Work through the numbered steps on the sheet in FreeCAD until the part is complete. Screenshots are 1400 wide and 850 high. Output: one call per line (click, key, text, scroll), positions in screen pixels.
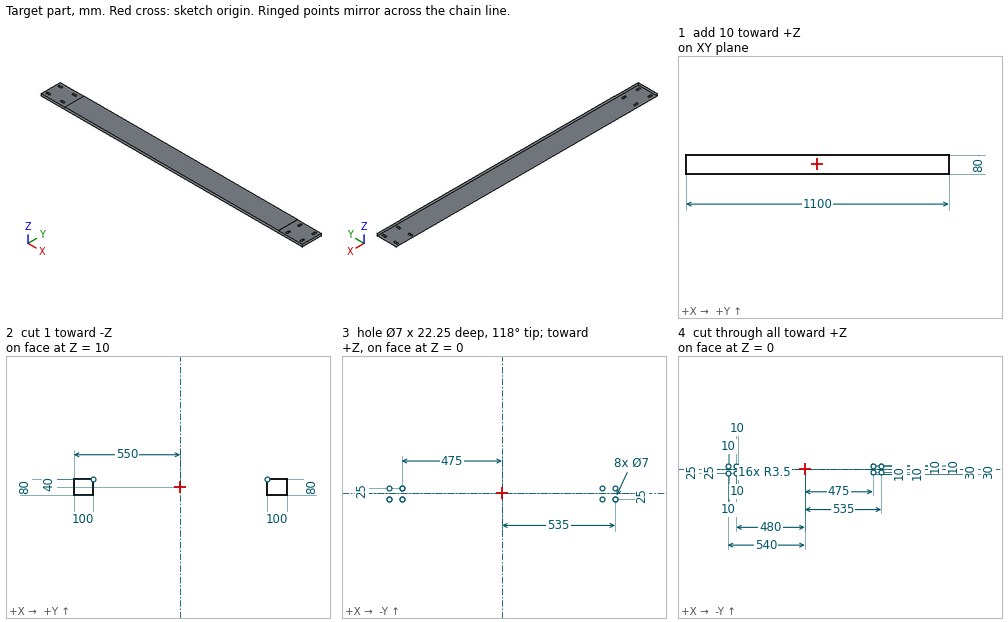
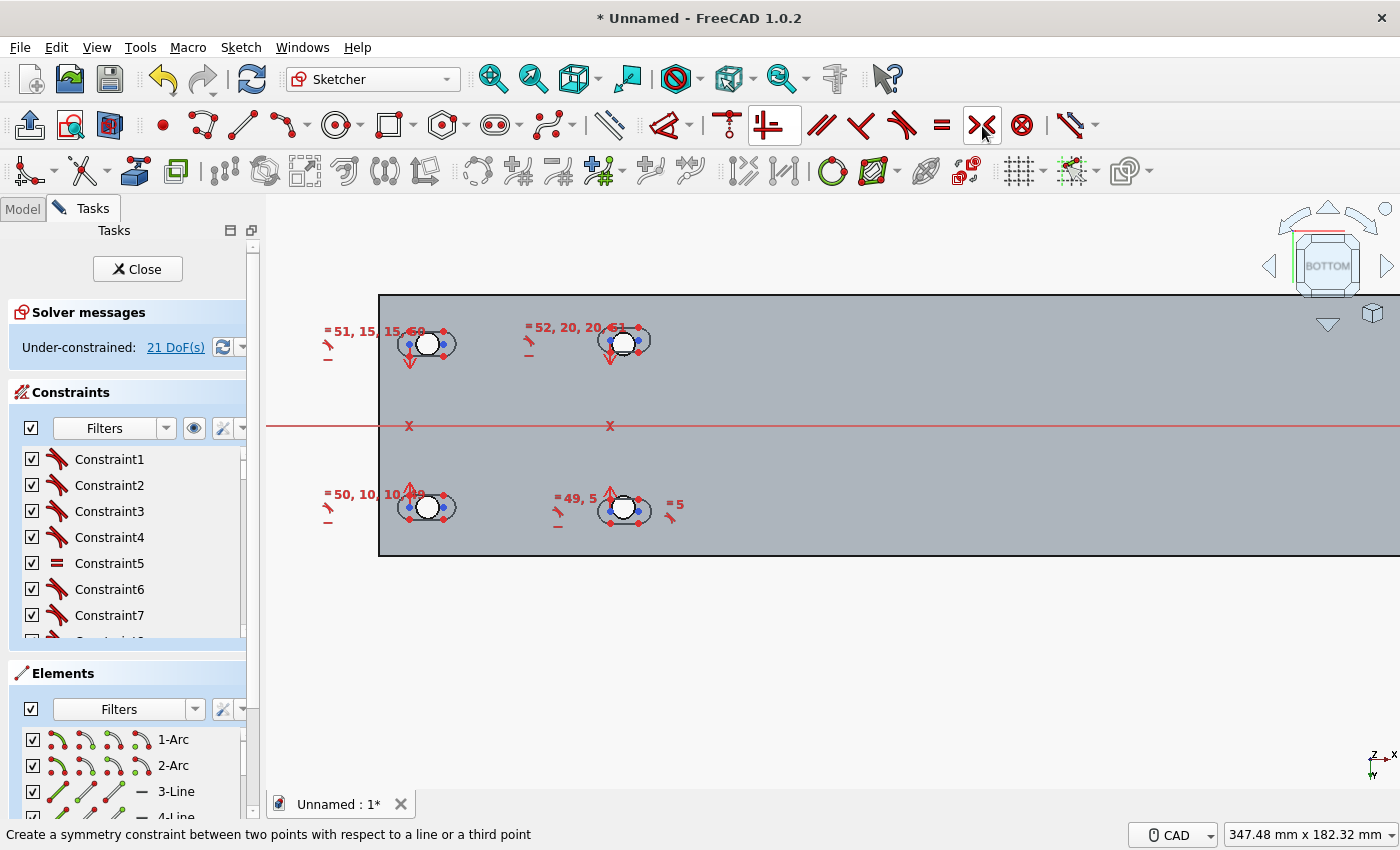
scroll(410, 508, down, 8)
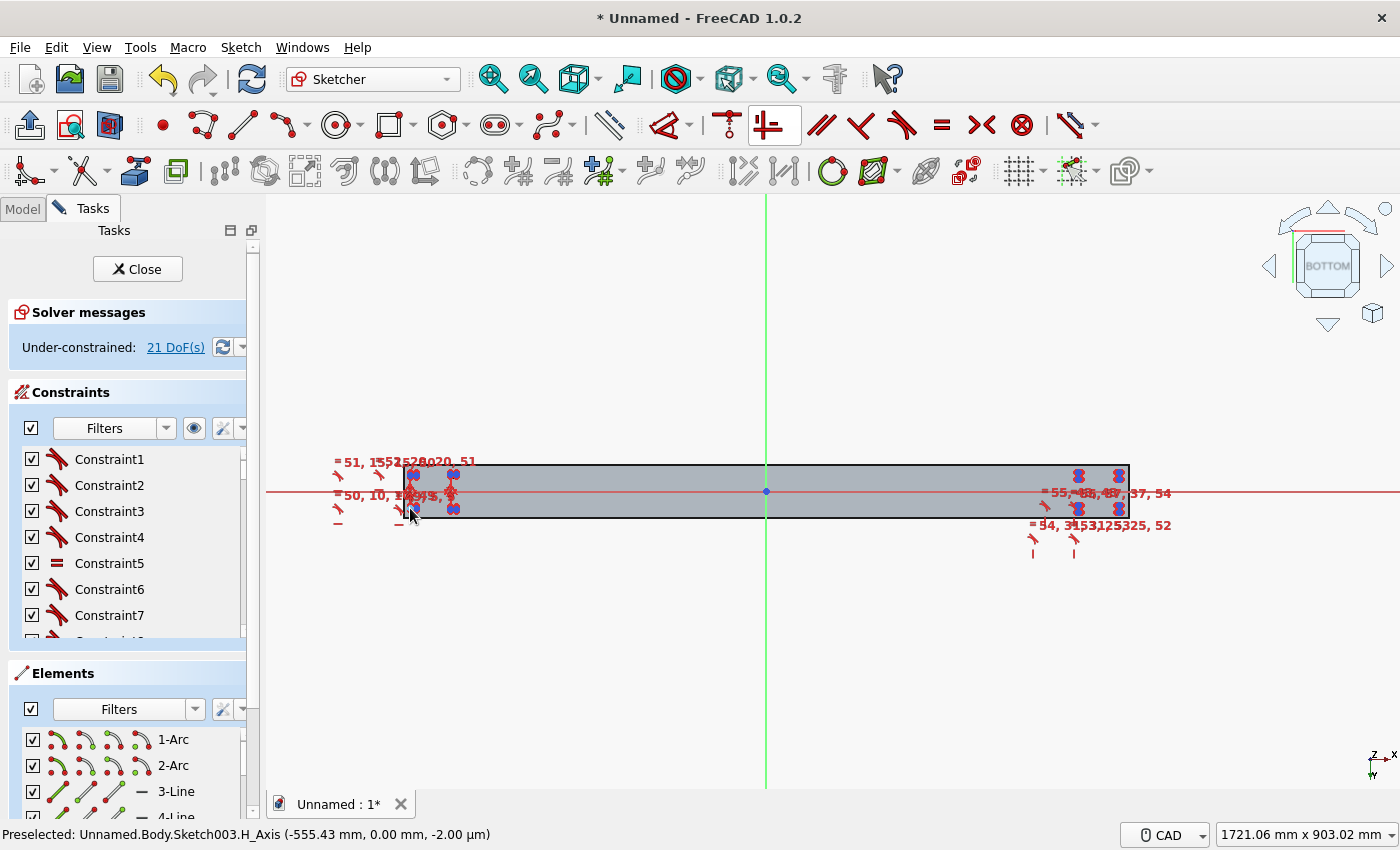
scroll(1119, 505, up, 8)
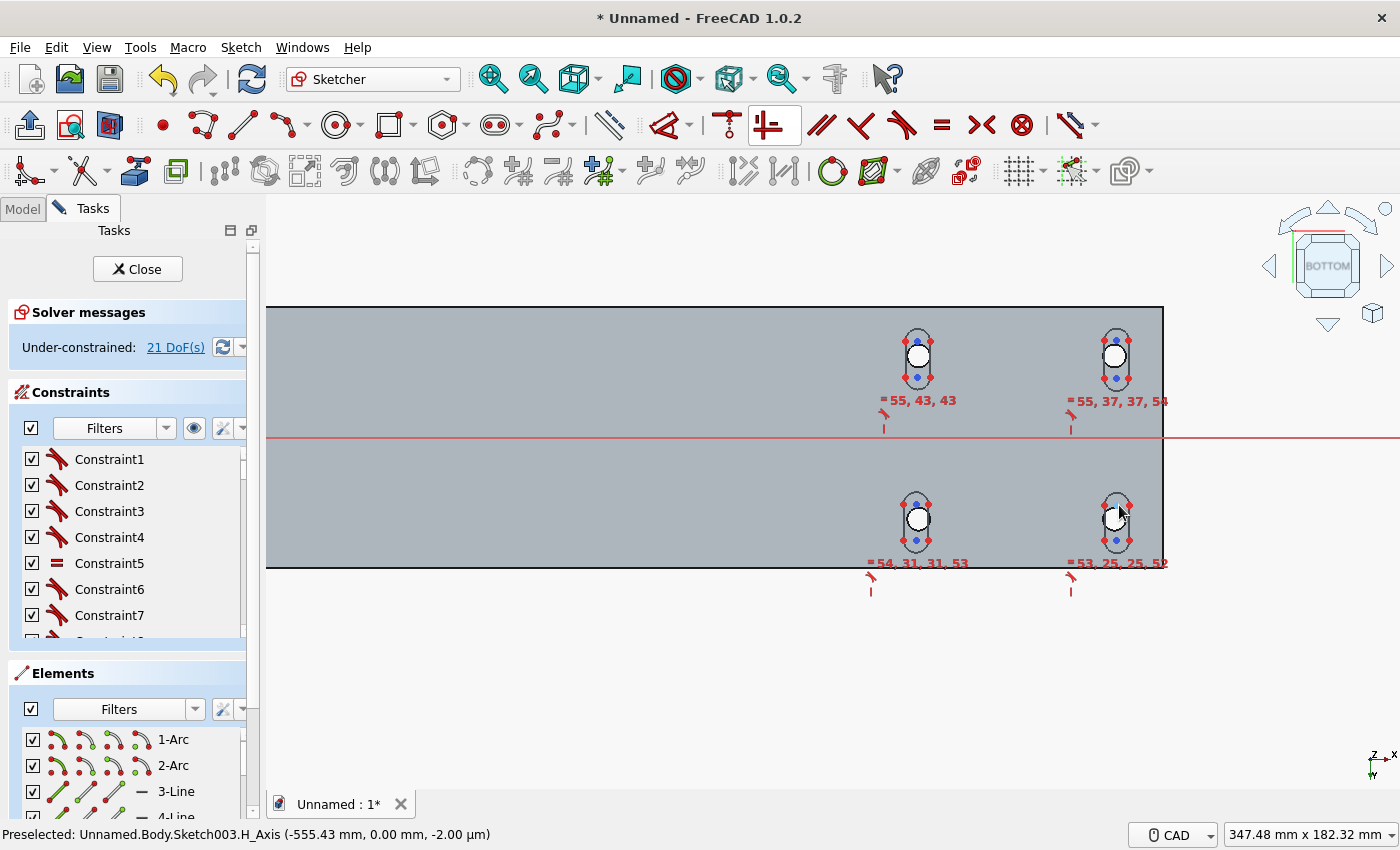
click(1117, 505)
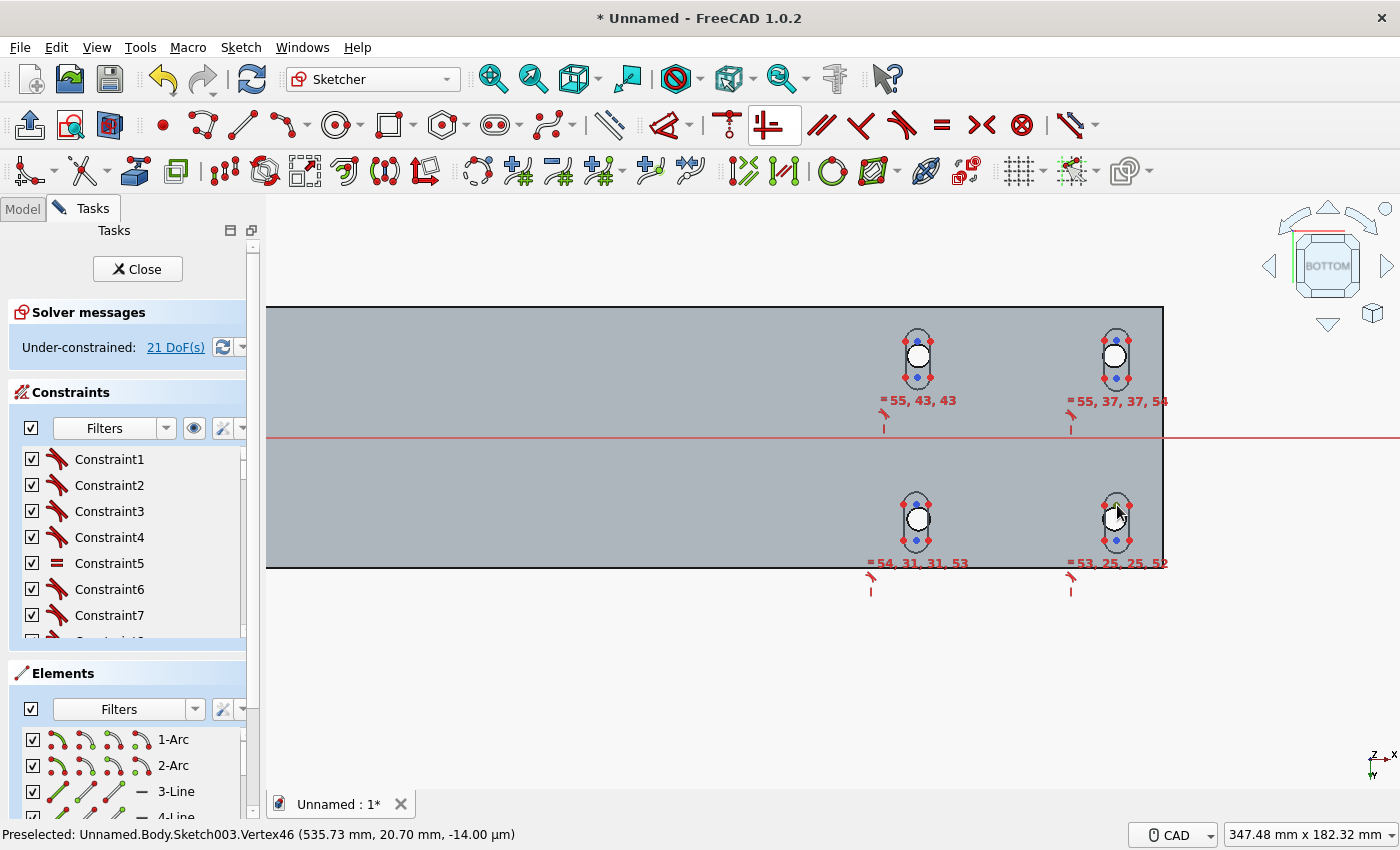
click(1117, 379)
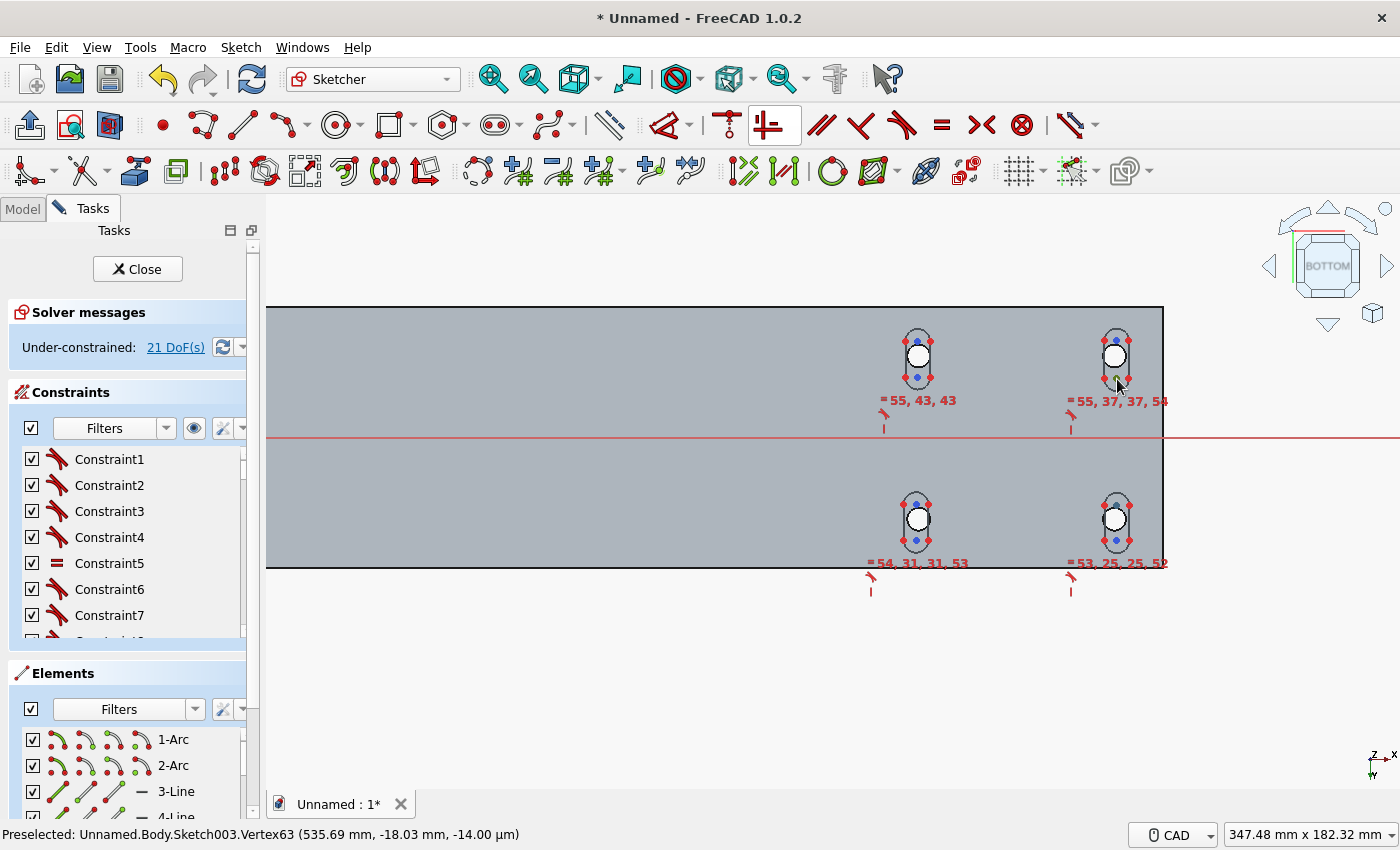
click(361, 438)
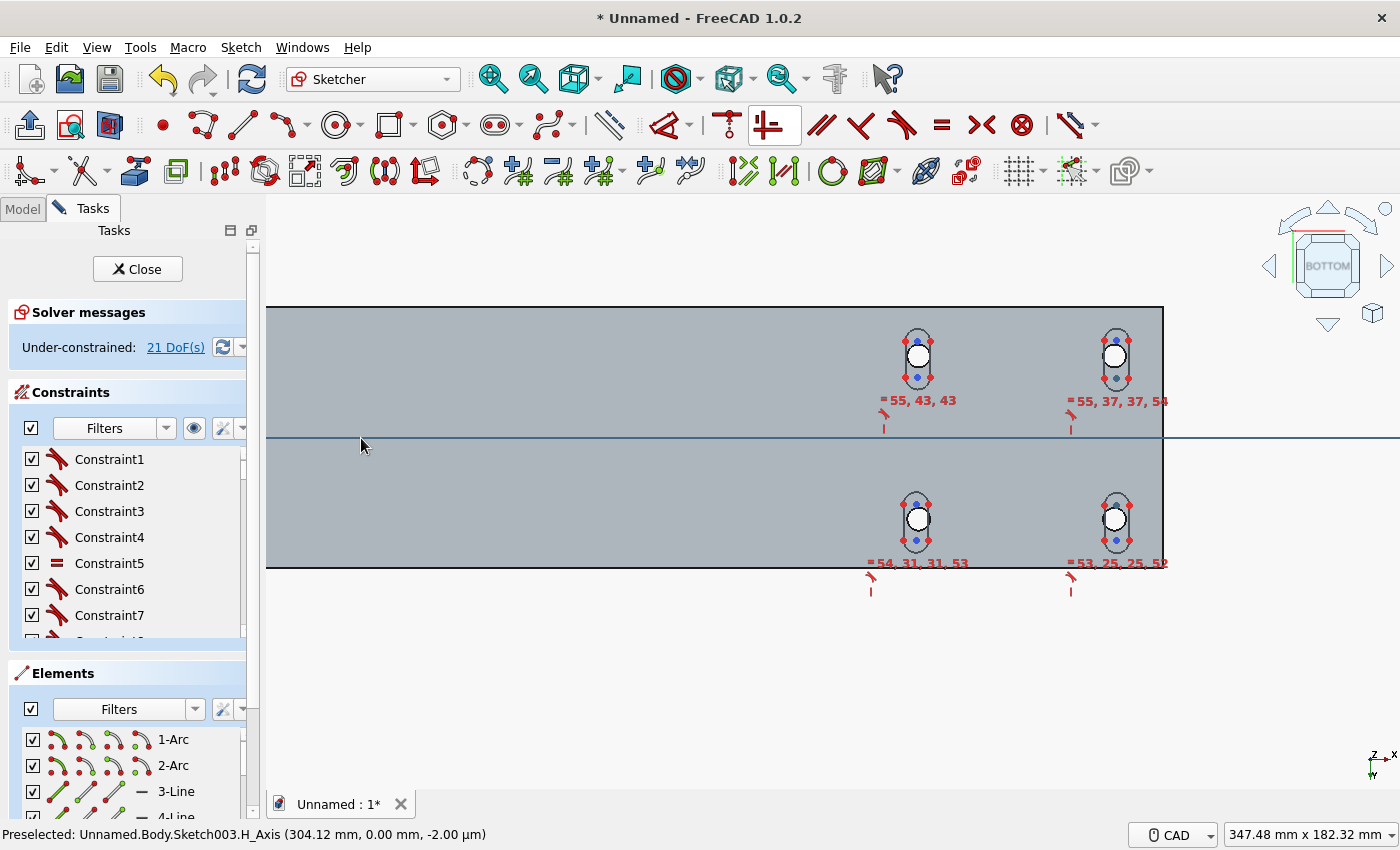
key(s)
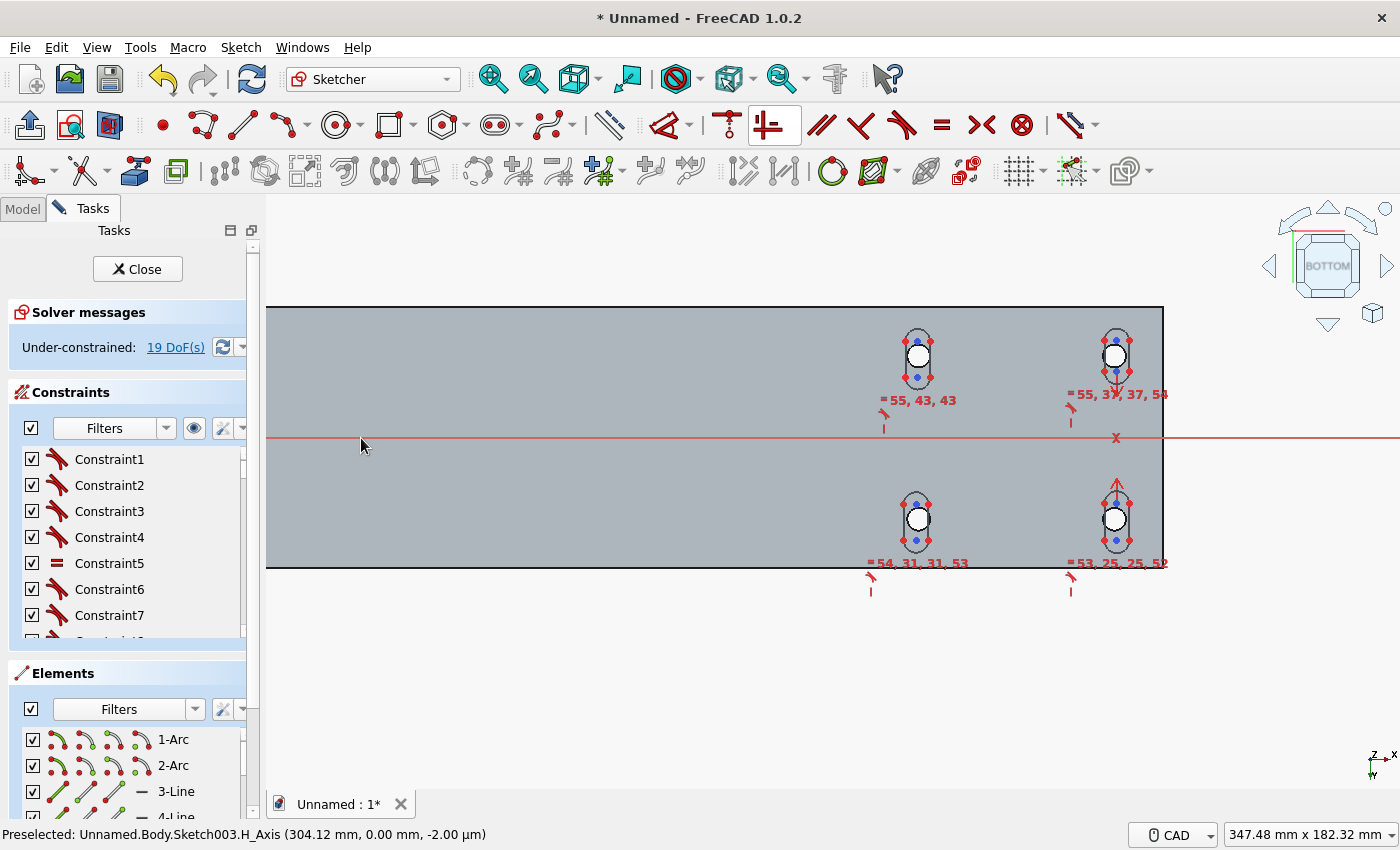
click(916, 505)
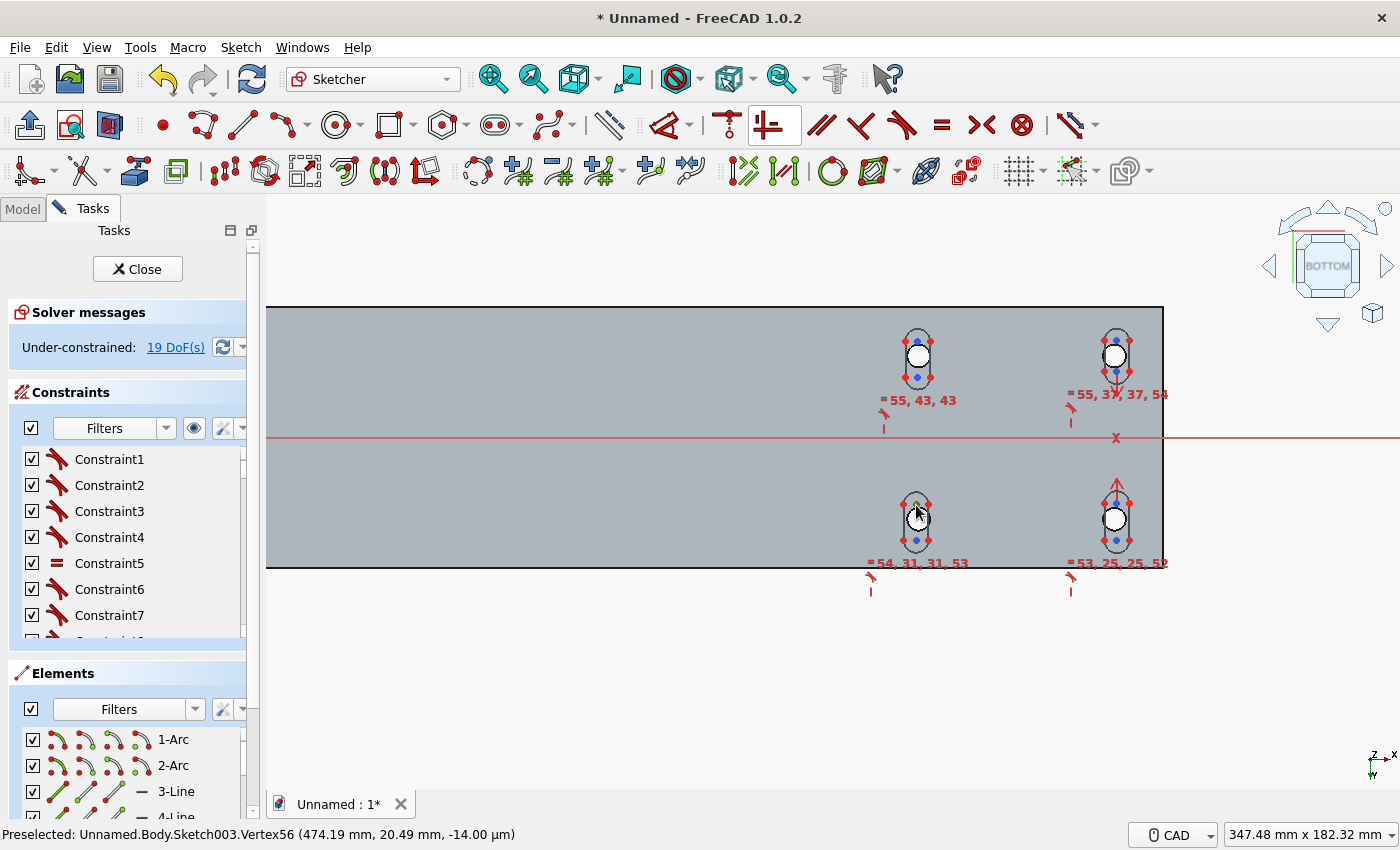
click(918, 377)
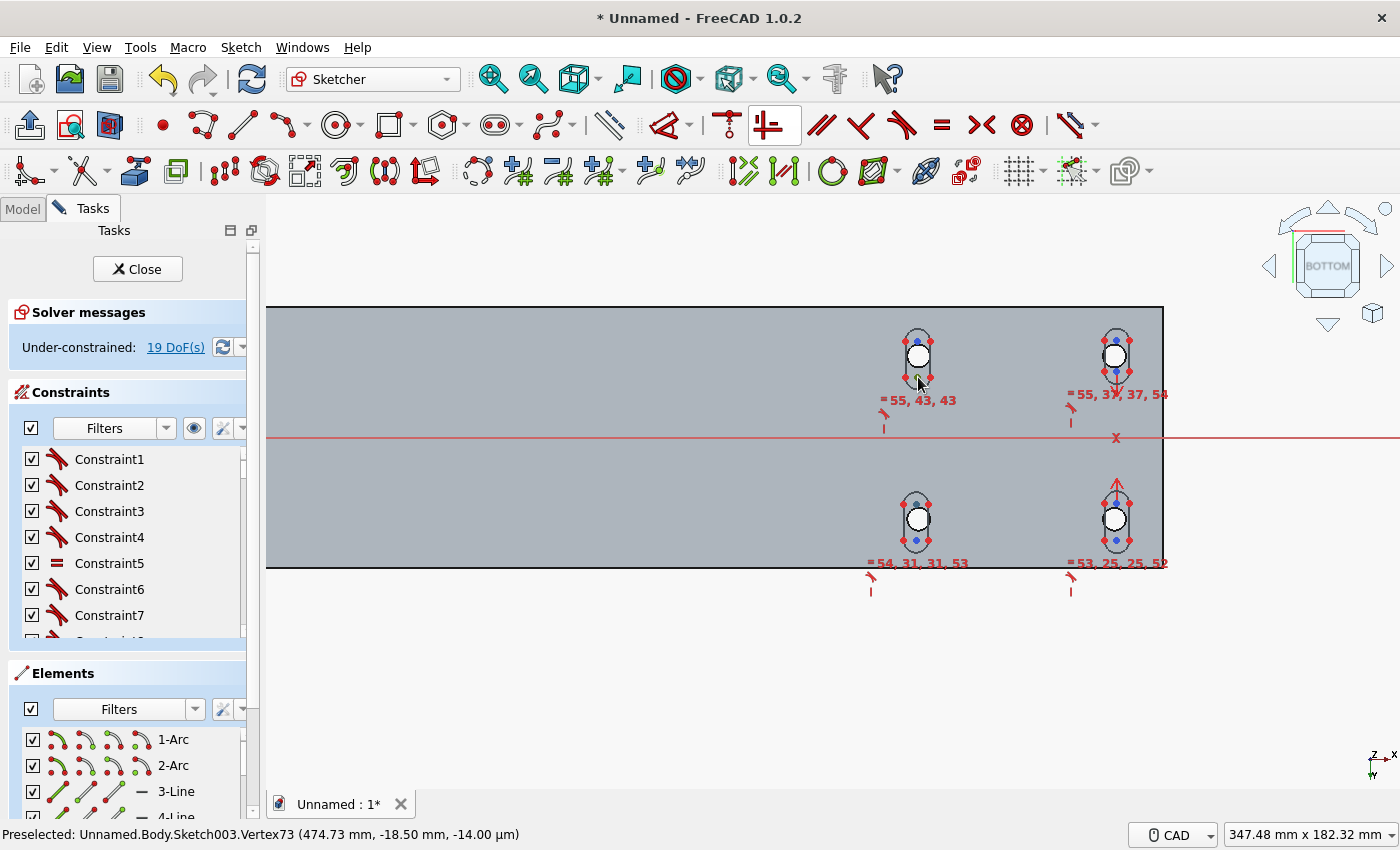
click(361, 438)